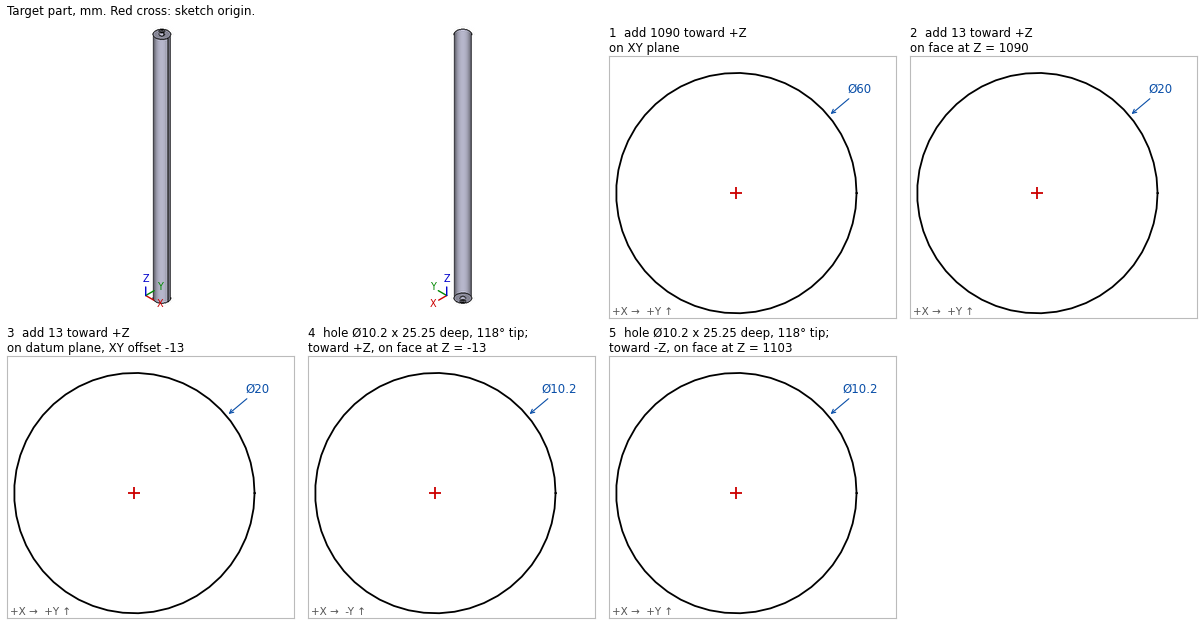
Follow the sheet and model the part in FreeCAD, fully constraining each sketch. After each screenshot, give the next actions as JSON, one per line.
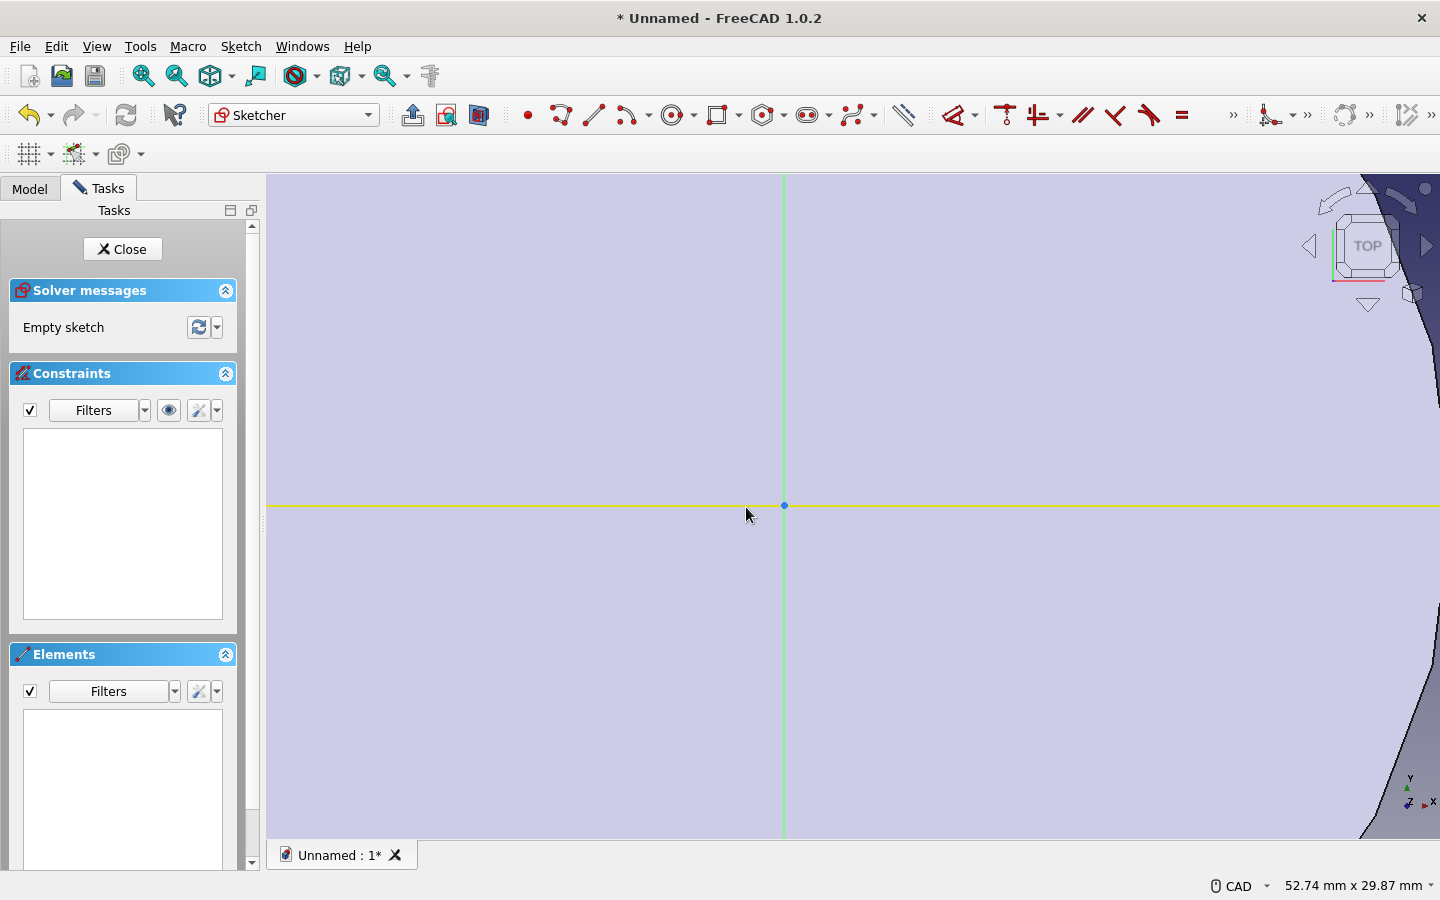
{"action": "left_click", "coordinate": [672, 116]}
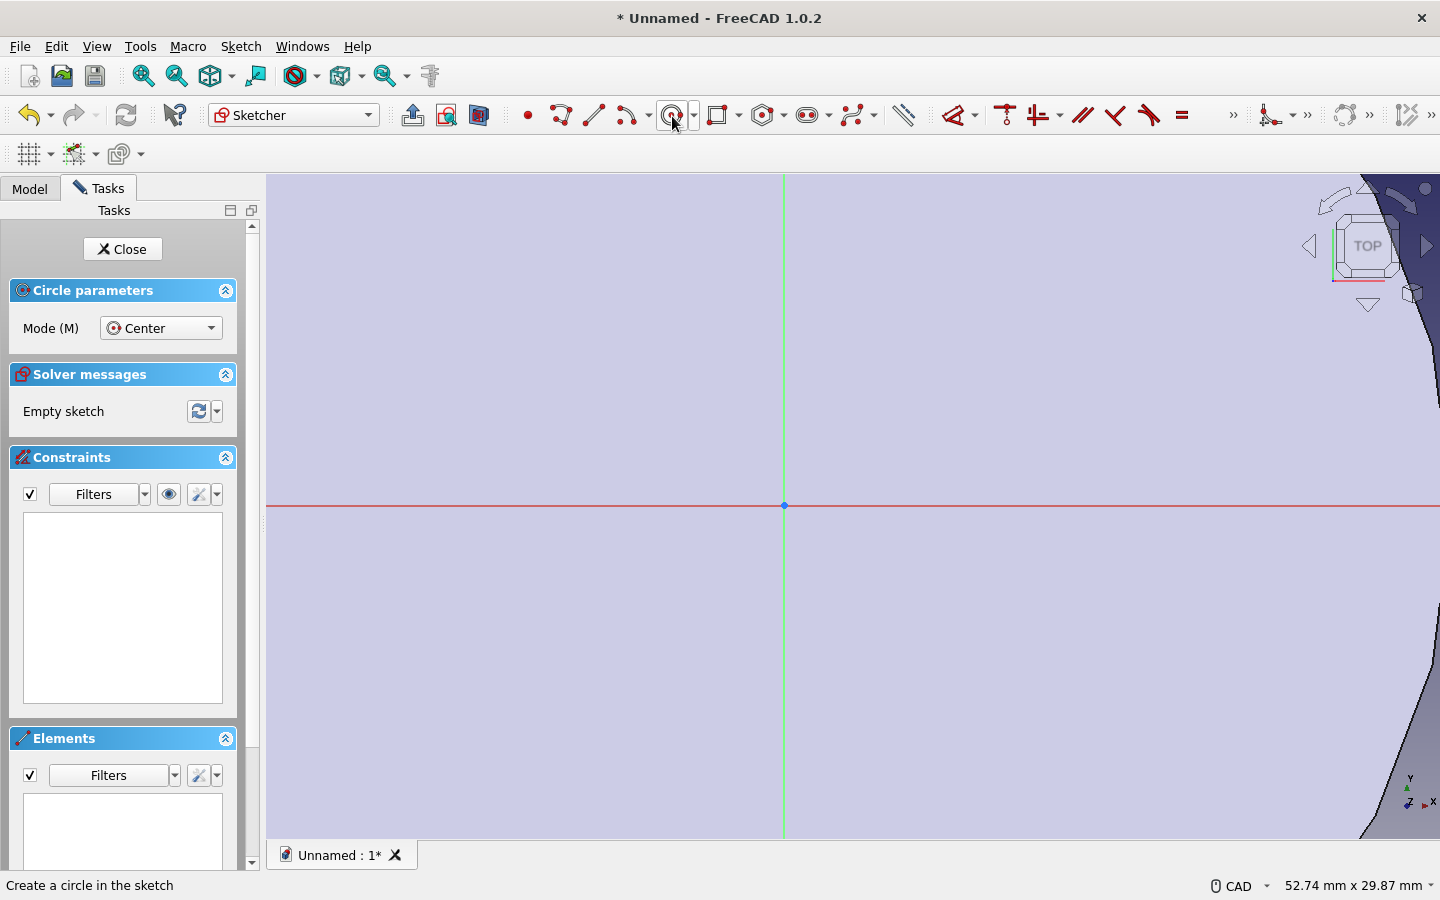
{"action": "left_click", "coordinate": [784, 506]}
{"action": "mouse_move", "coordinate": [941, 348]}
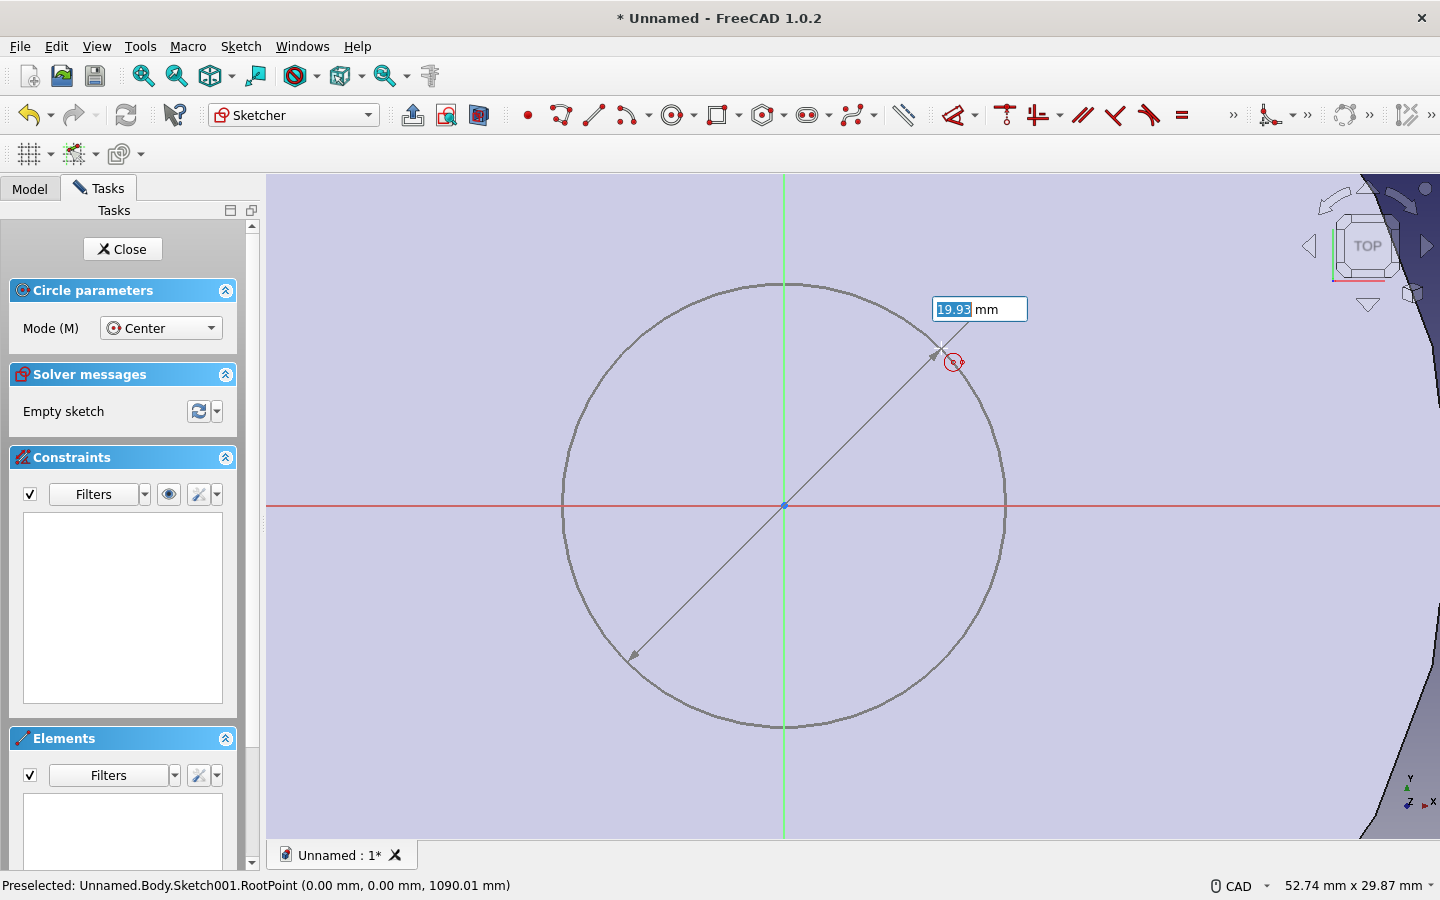
{"action": "type", "text": "20"}
{"action": "key", "text": "Return"}
{"action": "key", "text": "Escape"}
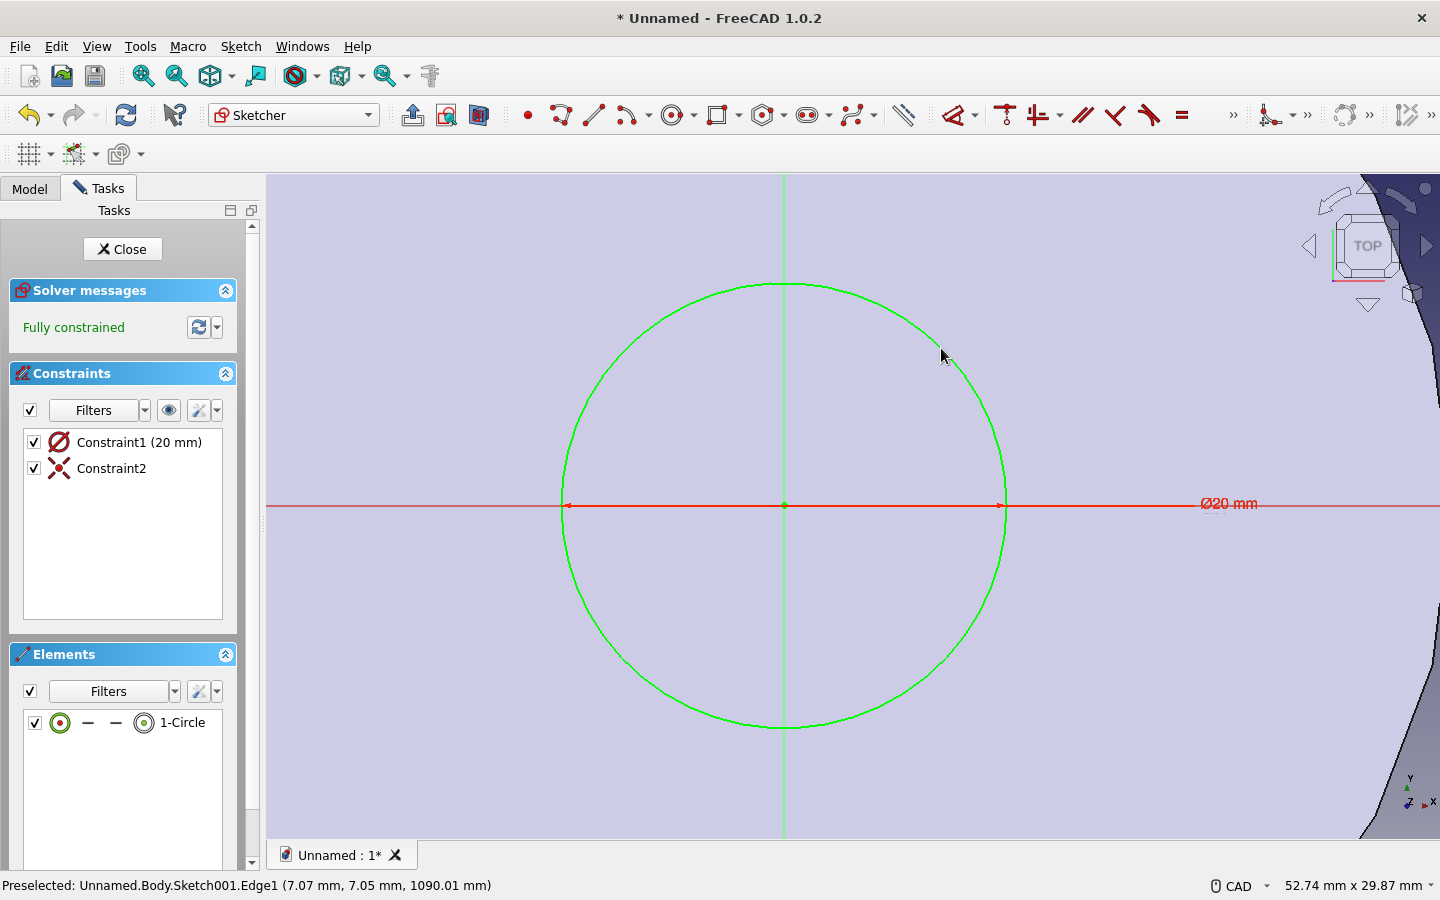
{"action": "left_click", "coordinate": [123, 249]}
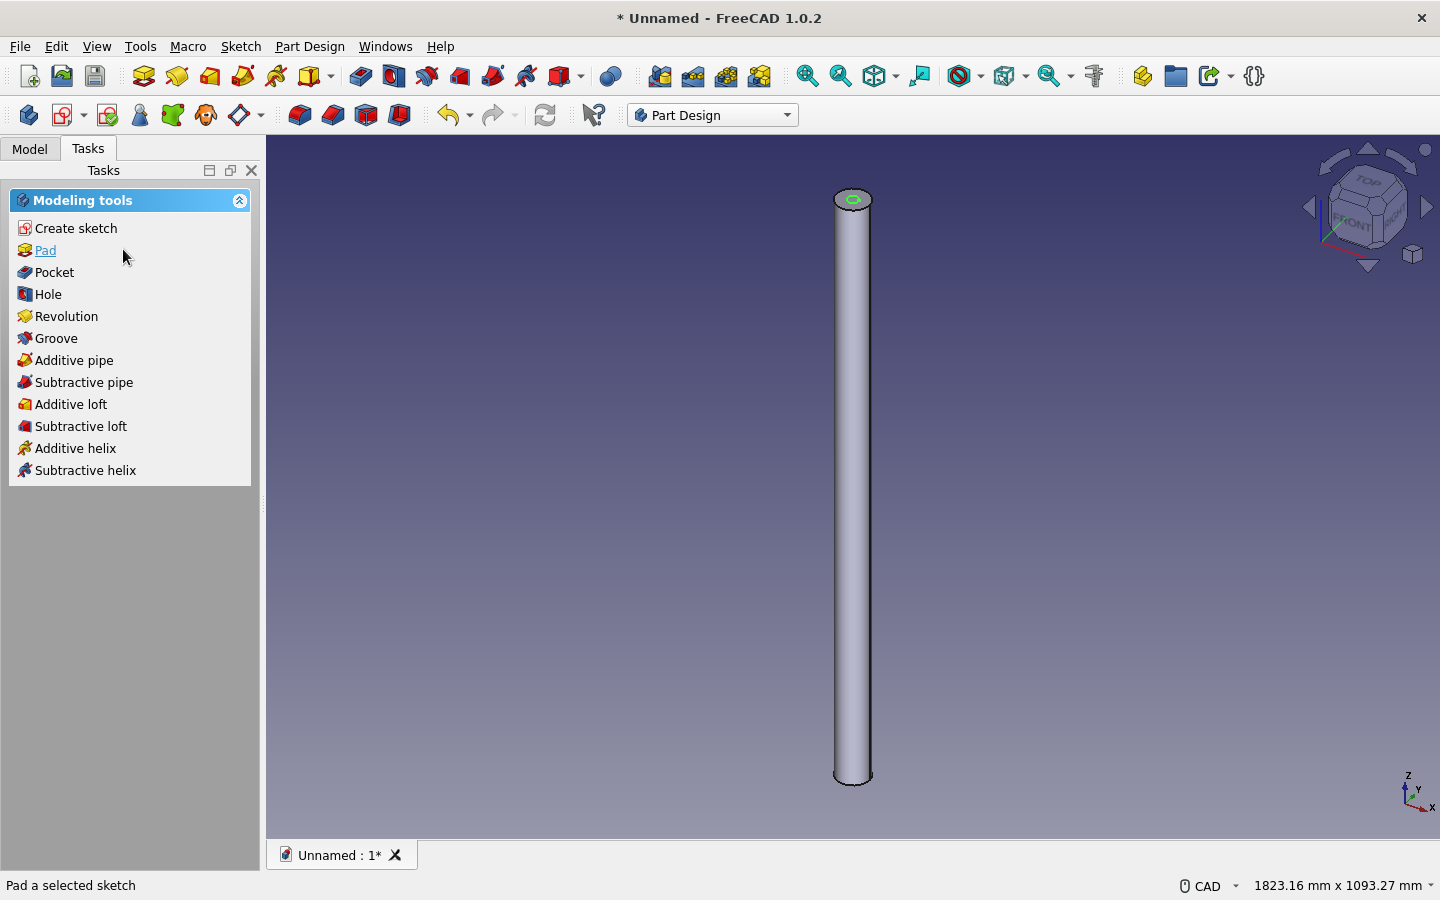
{"action": "left_click", "coordinate": [144, 76]}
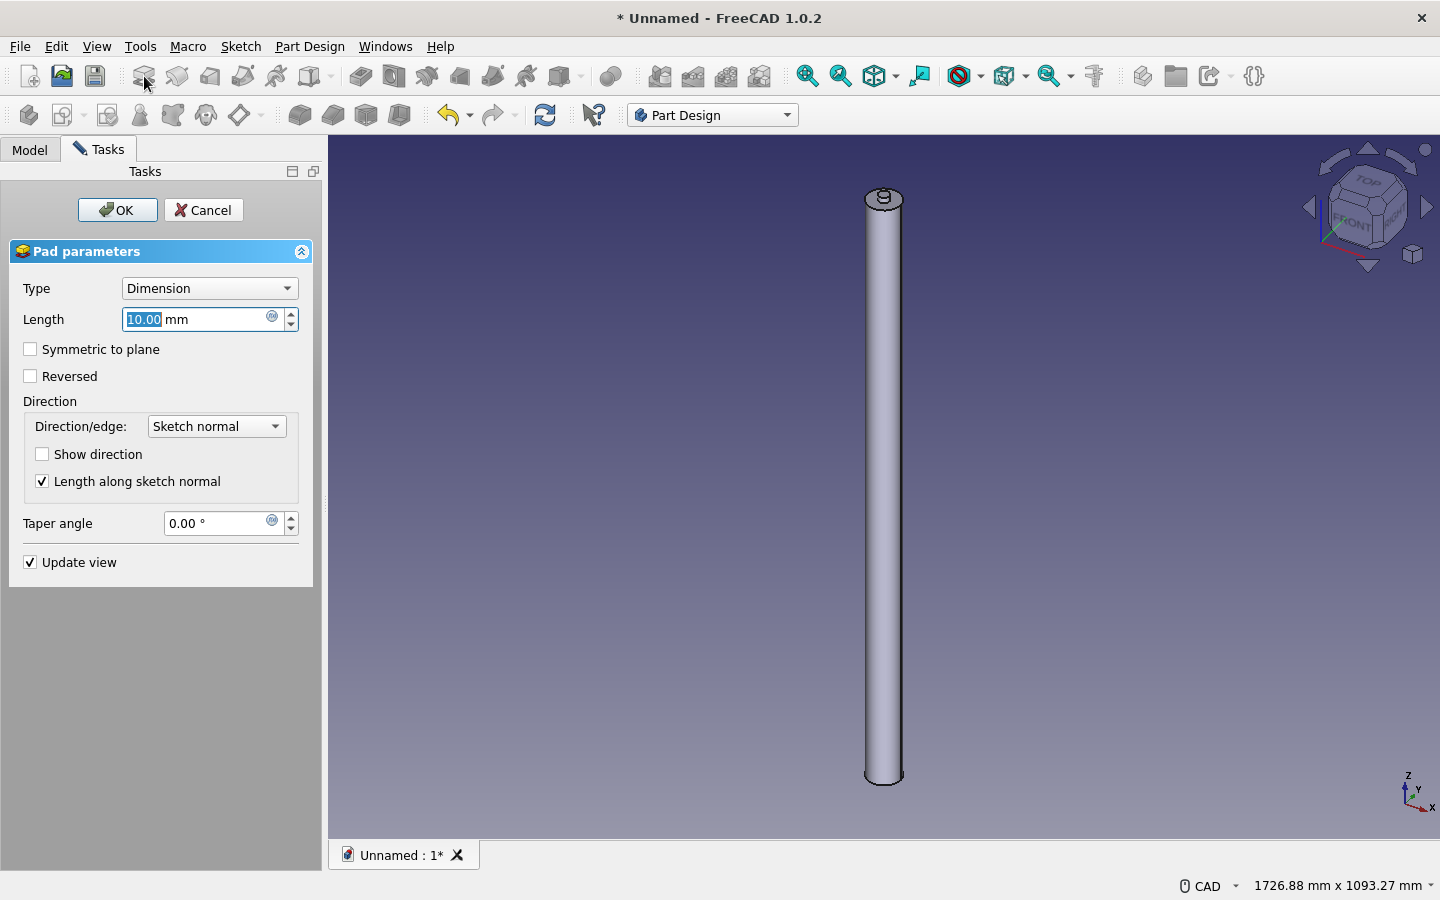
{"action": "type", "text": "13"}
{"action": "key", "text": "Tab"}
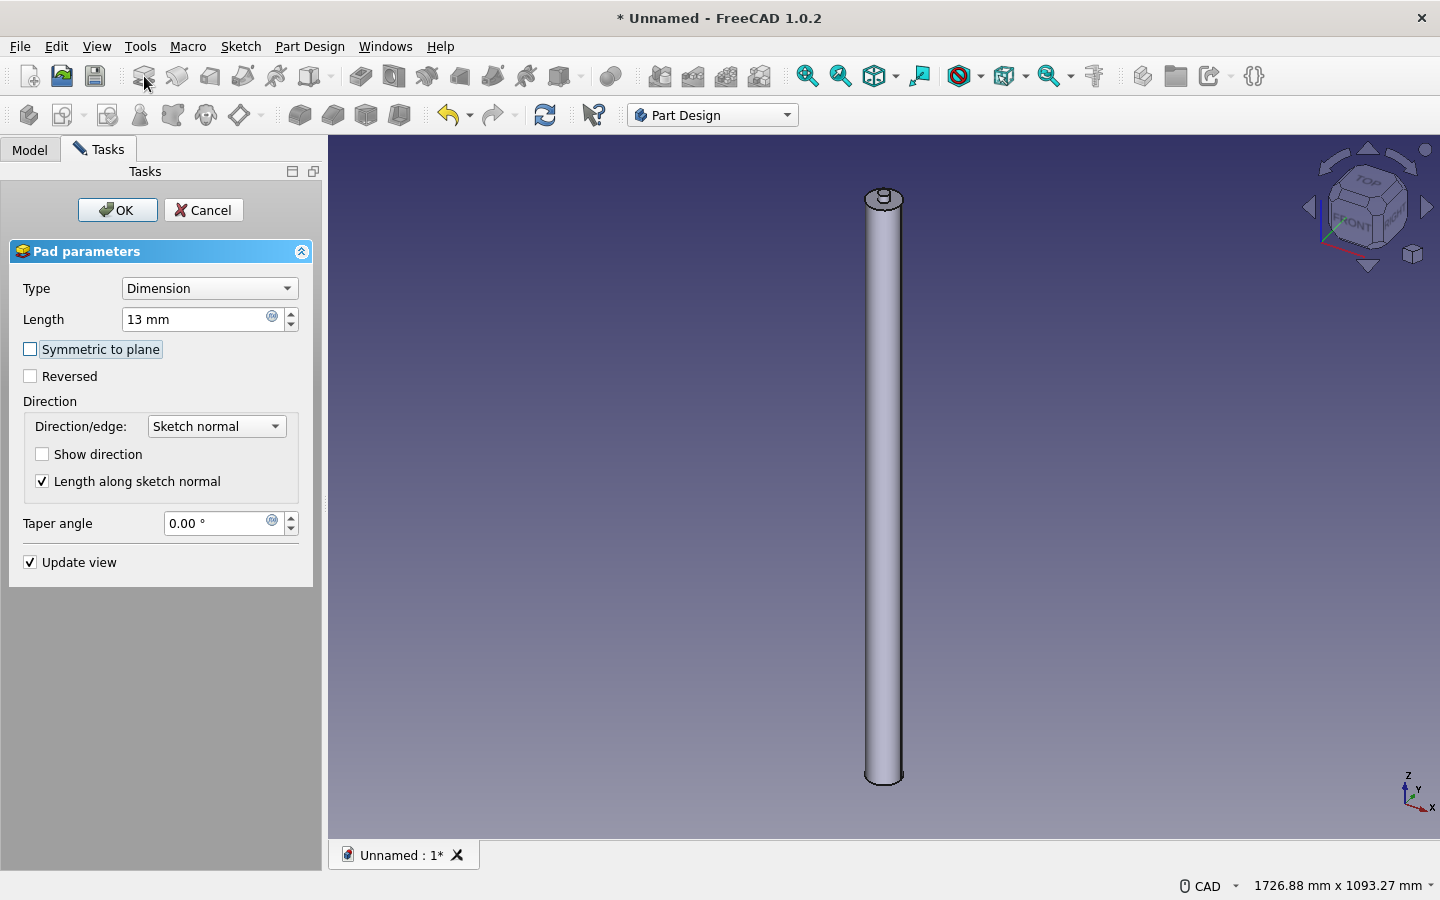
{"action": "left_click", "coordinate": [118, 210]}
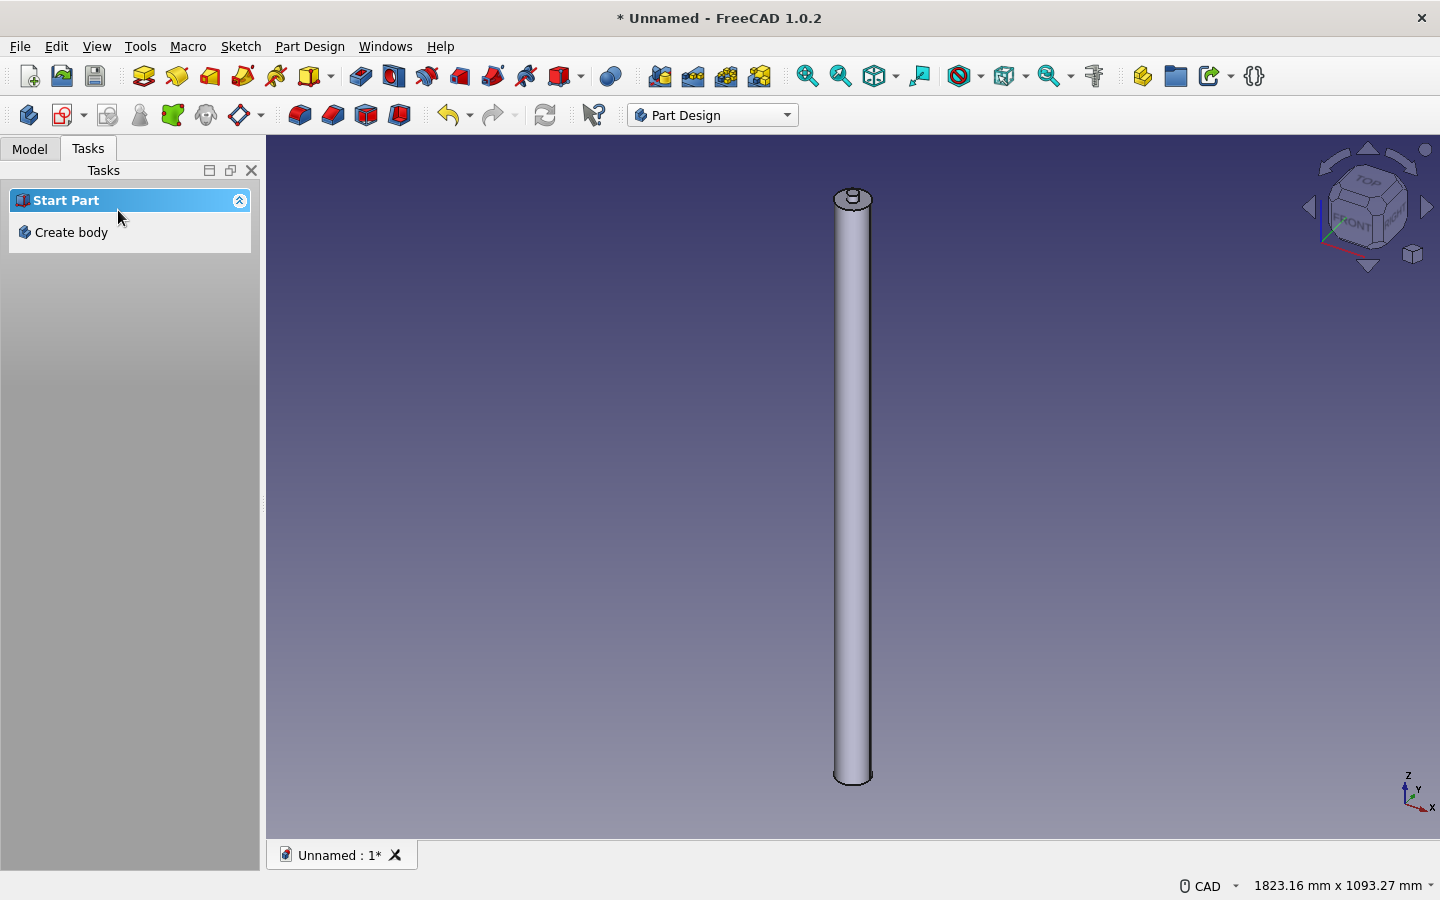
{"action": "left_click", "coordinate": [30, 148]}